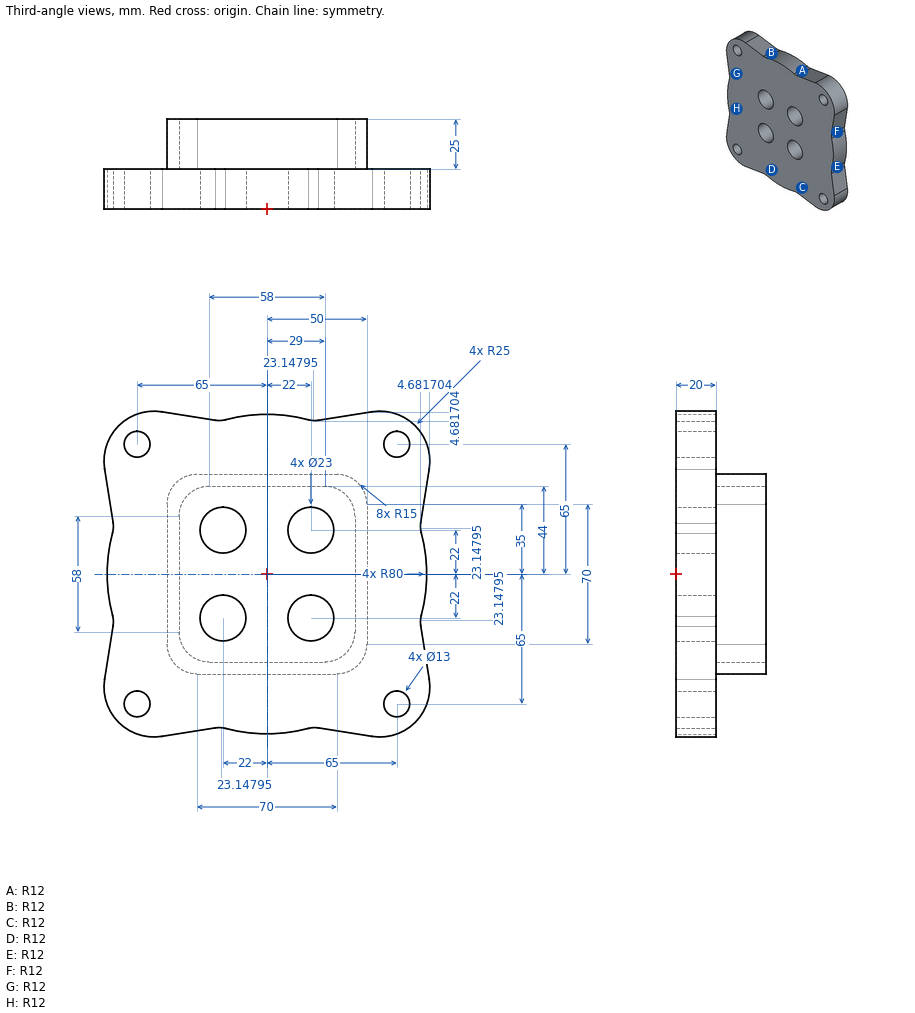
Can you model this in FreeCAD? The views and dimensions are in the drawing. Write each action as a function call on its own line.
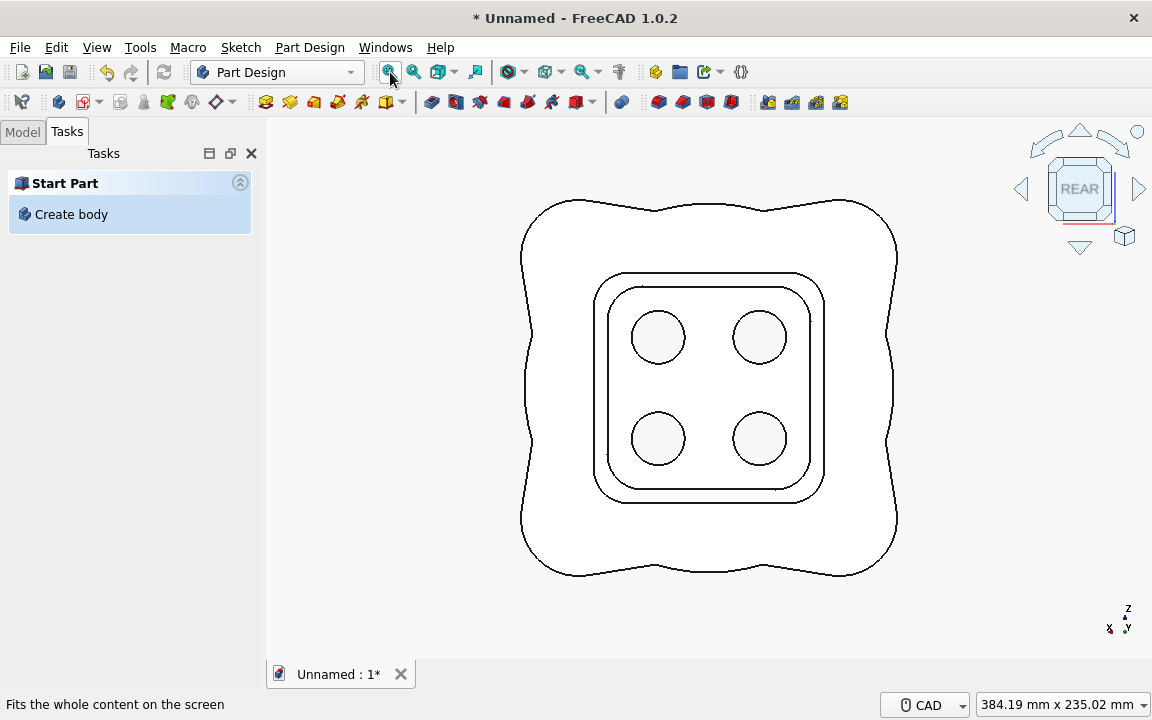
key(6)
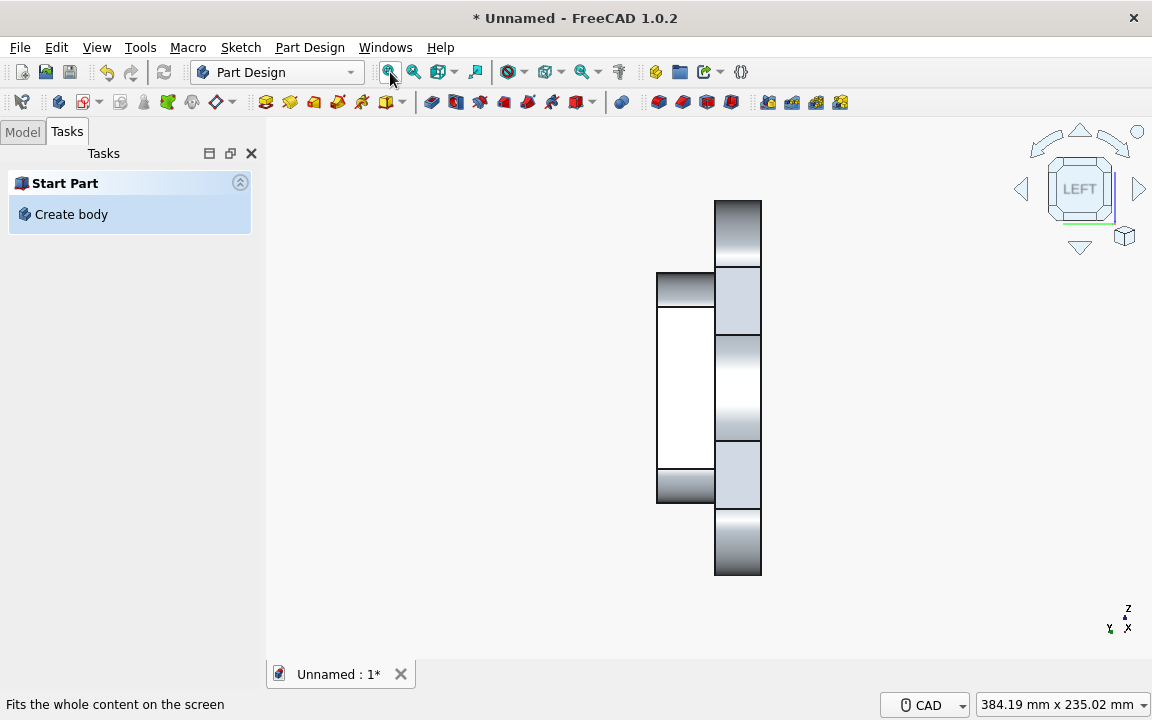
key(v)
key(3)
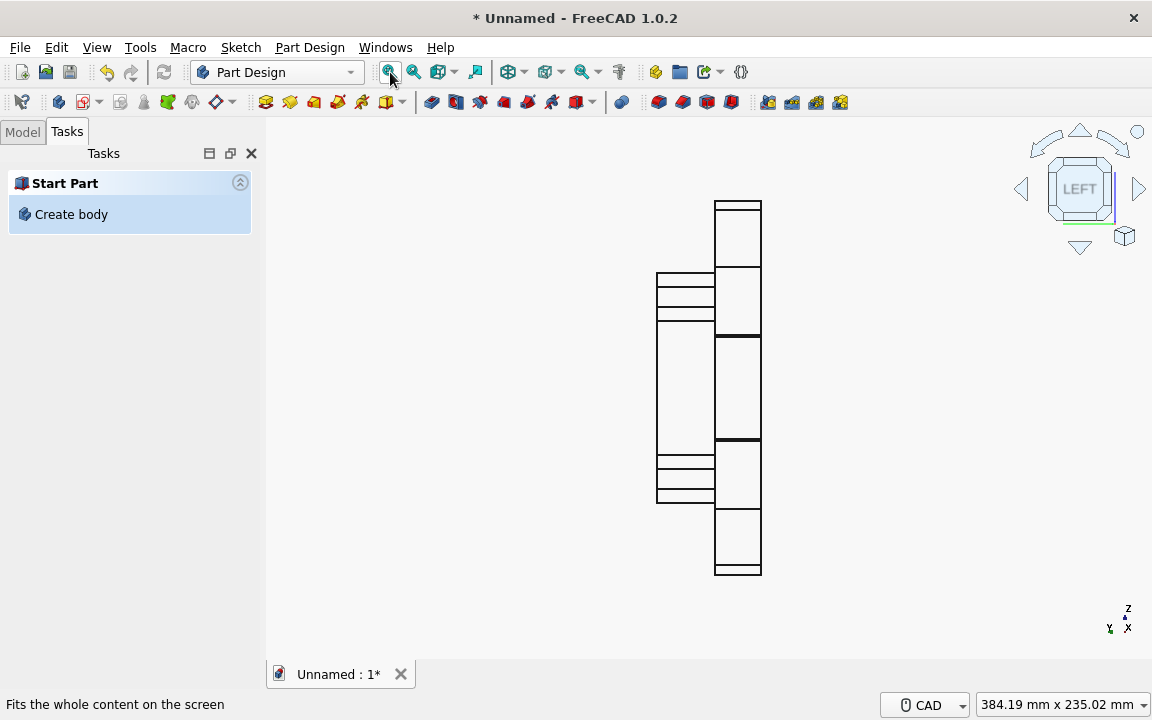
key(0)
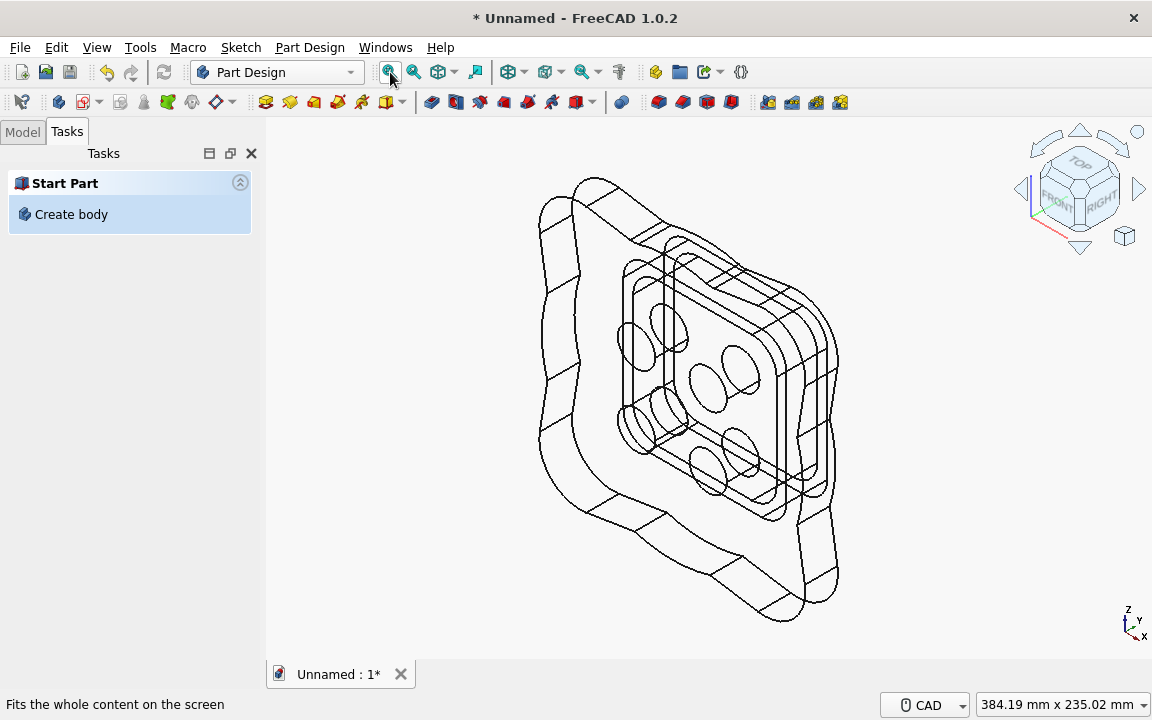
click(726, 565)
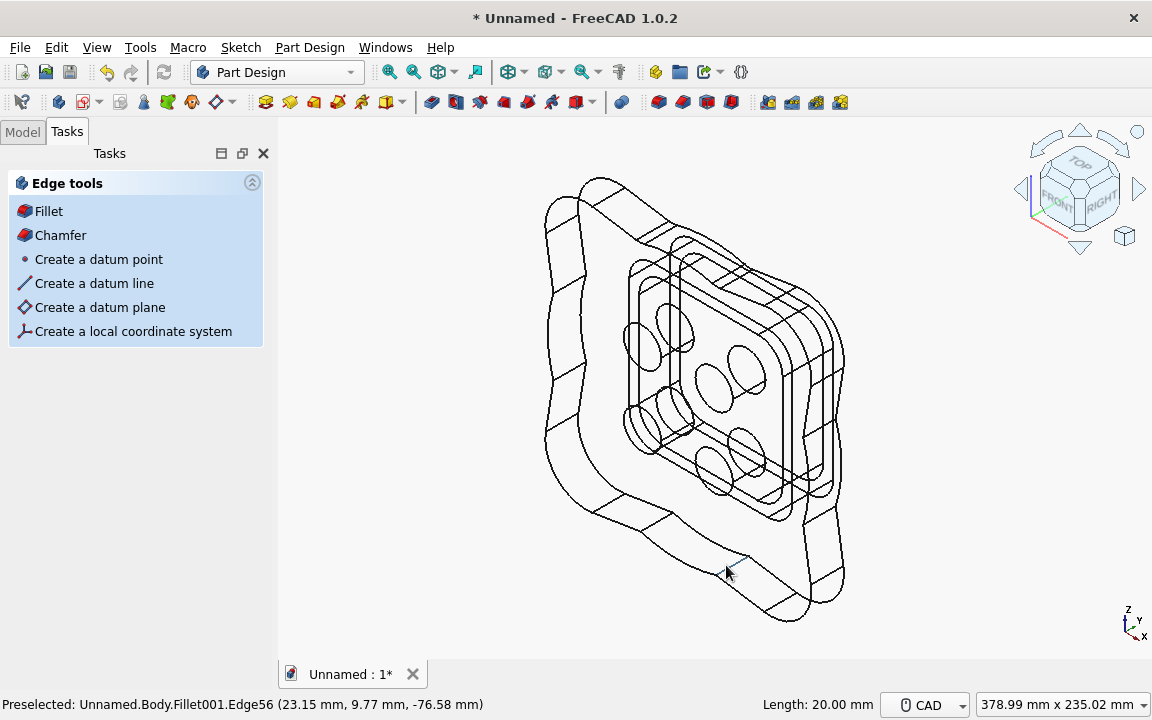
key(v)
key(1)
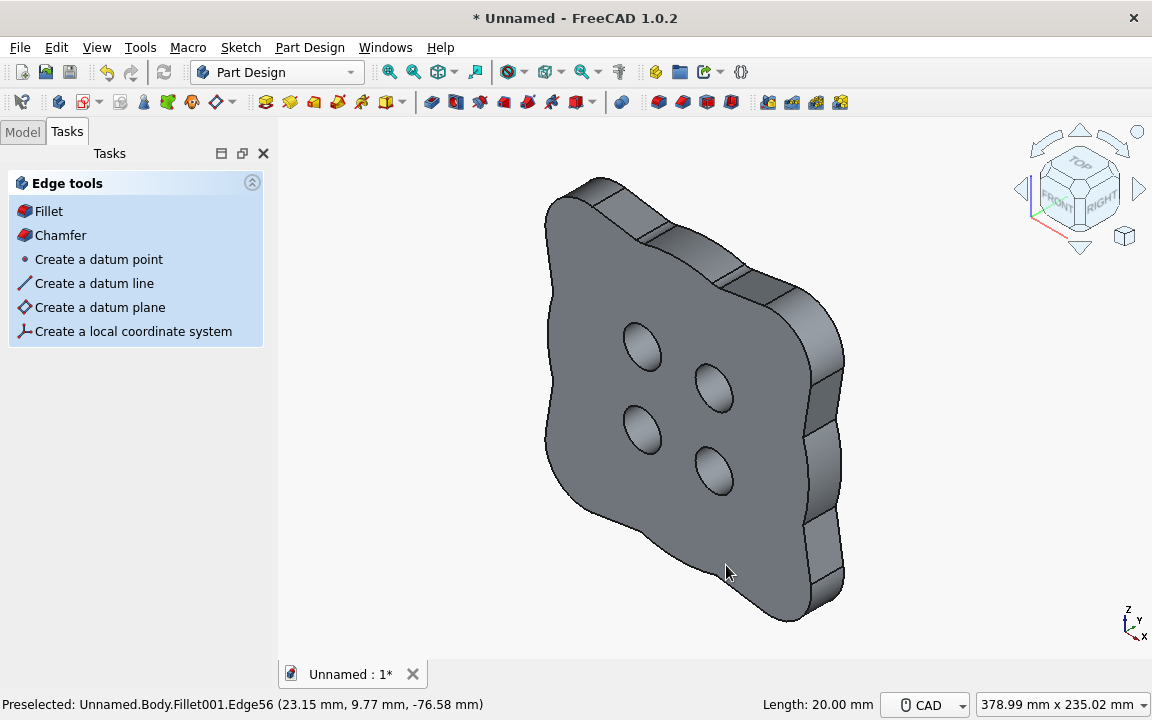
click(660, 102)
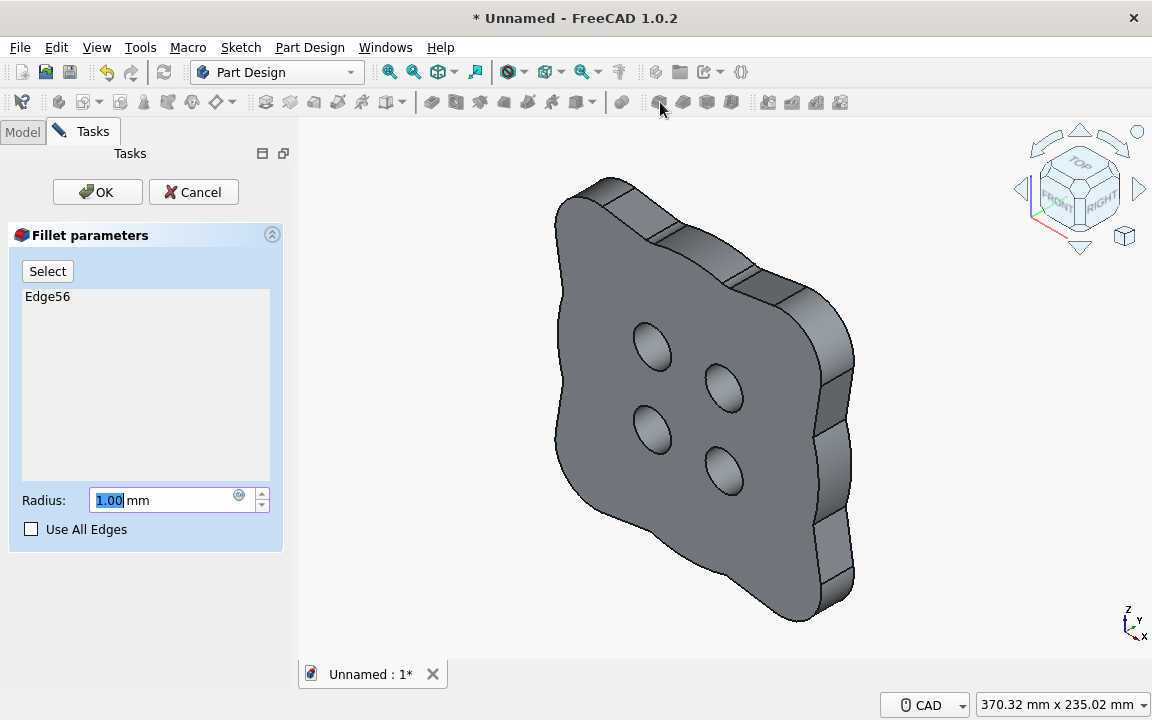
text(12)
key(Tab)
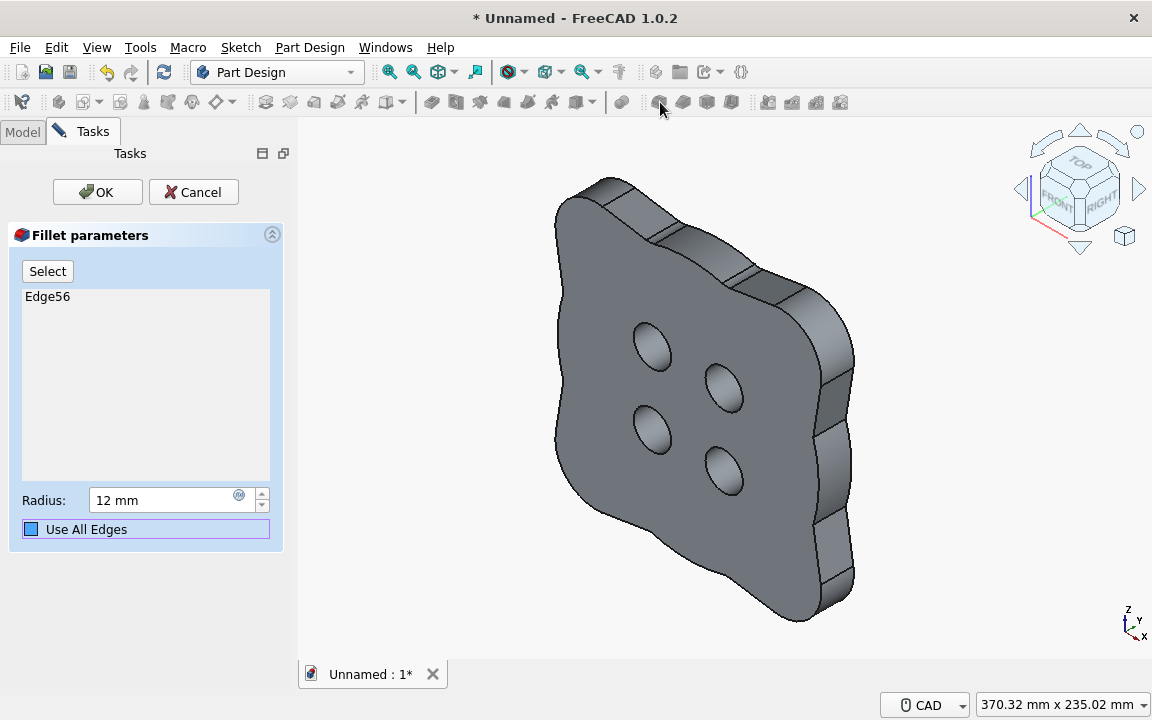
click(98, 192)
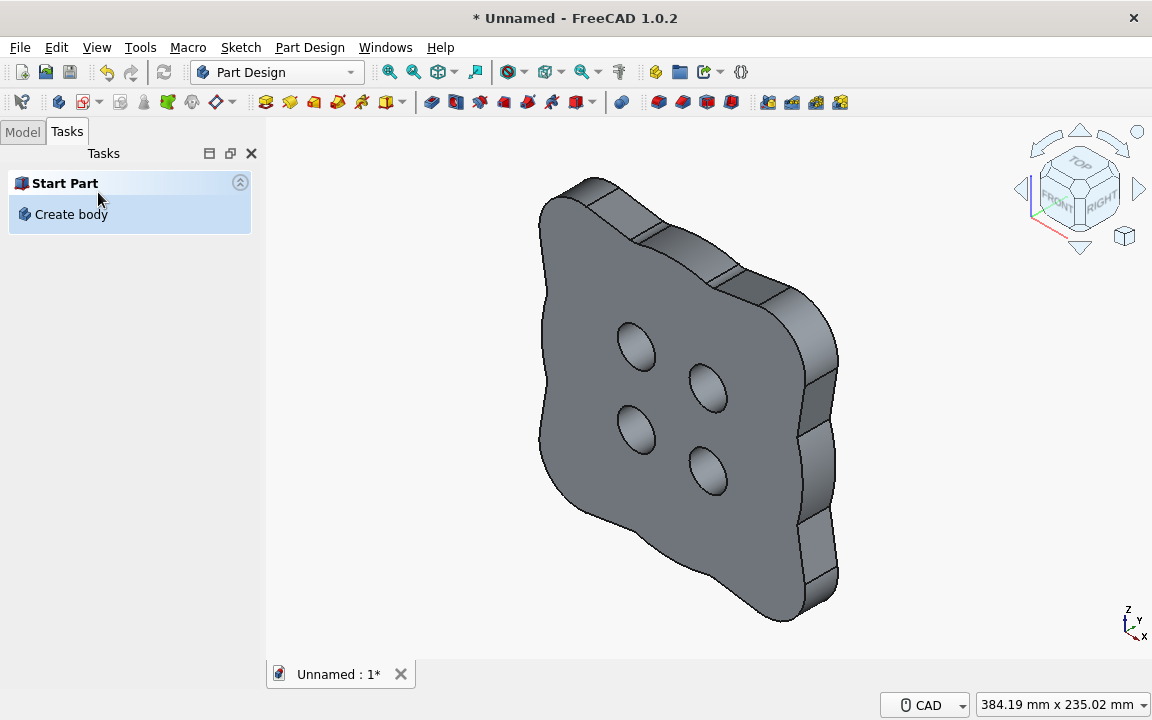
key(2)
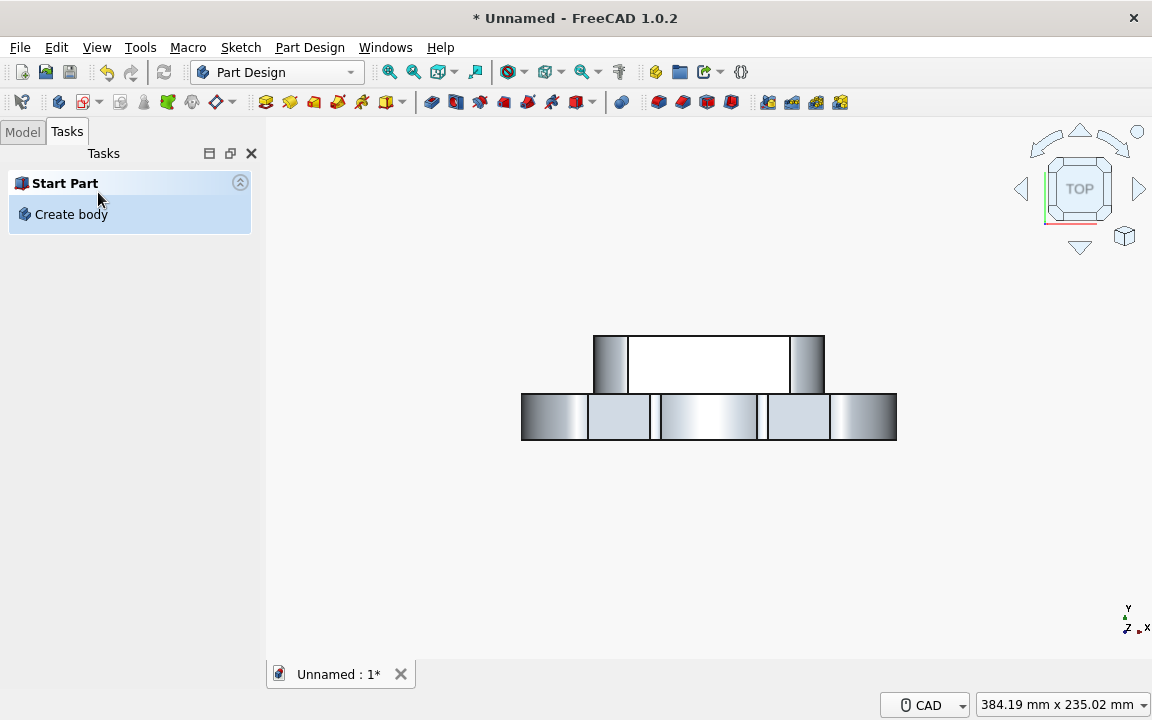
click(390, 72)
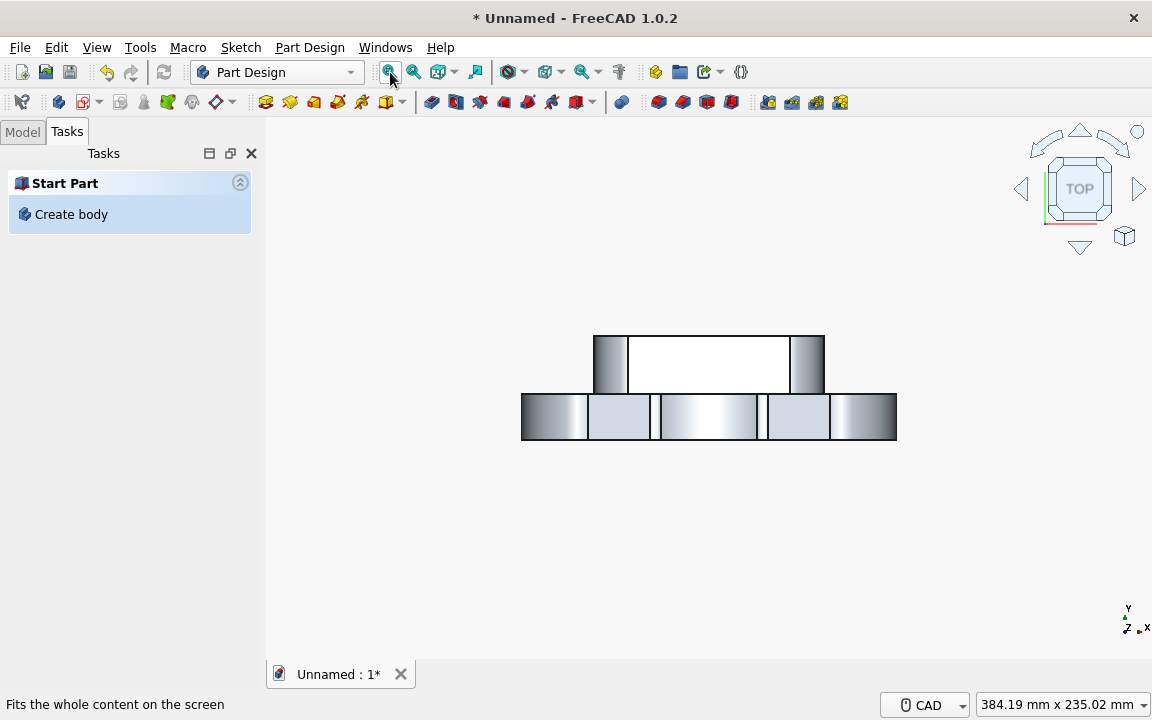
key(0)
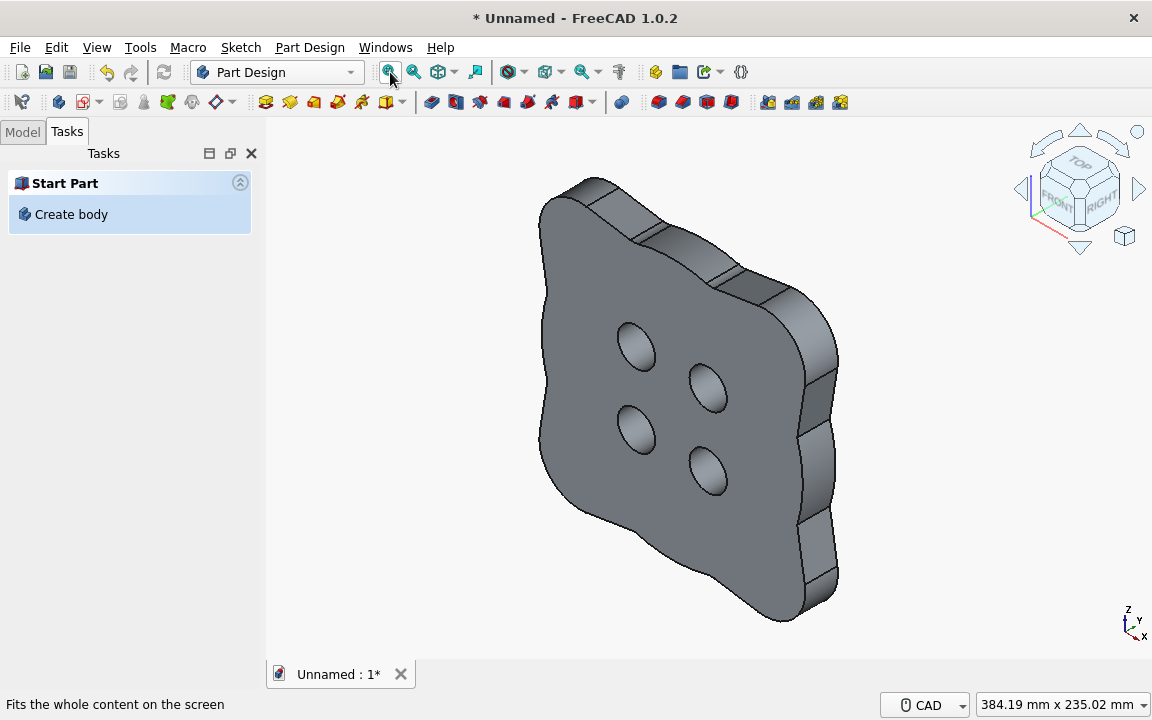
key(1)